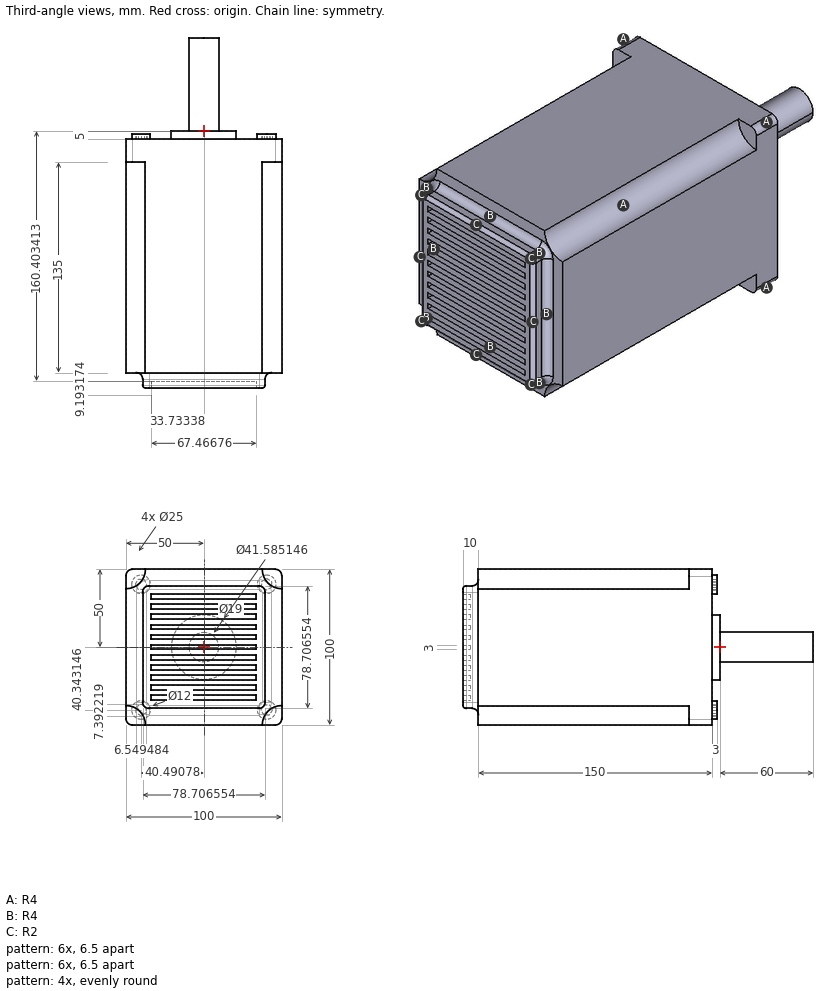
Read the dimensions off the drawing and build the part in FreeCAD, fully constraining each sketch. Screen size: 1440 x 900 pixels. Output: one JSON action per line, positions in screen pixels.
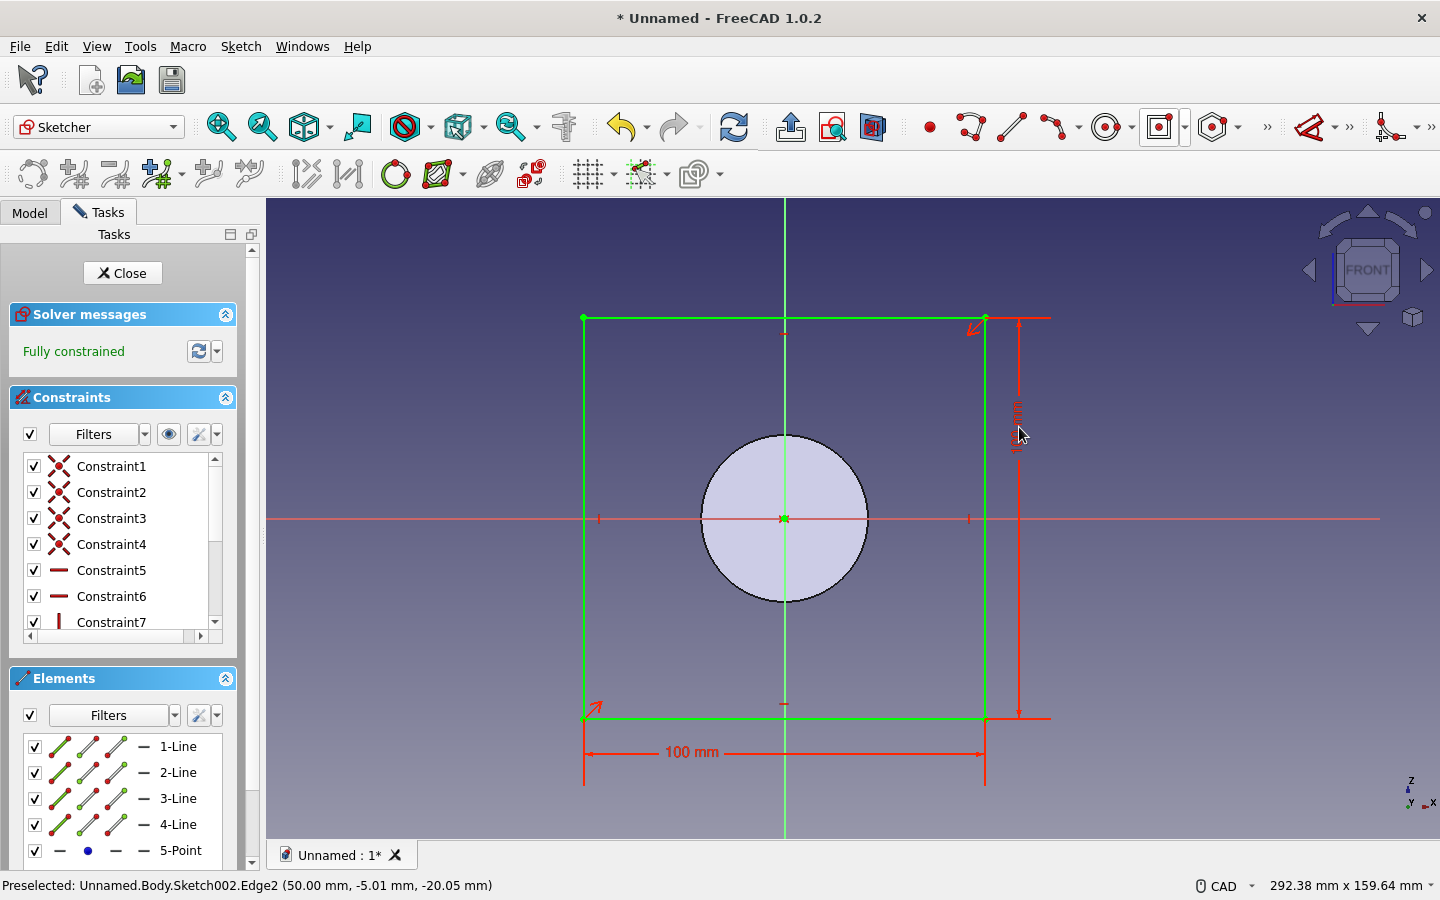
{"action": "left_click", "coordinate": [123, 273]}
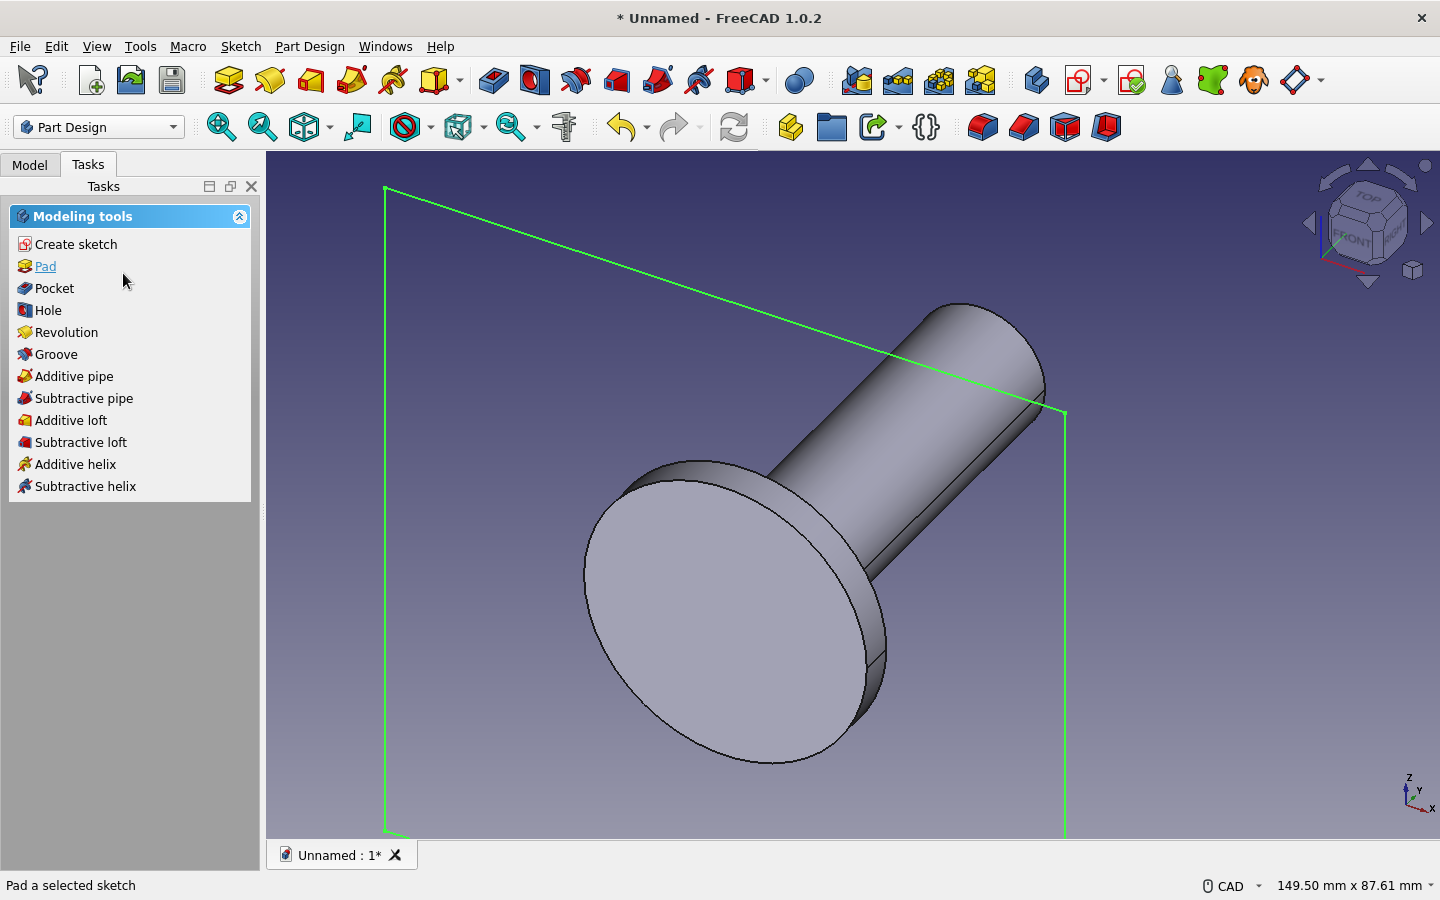
{"action": "left_click", "coordinate": [229, 80]}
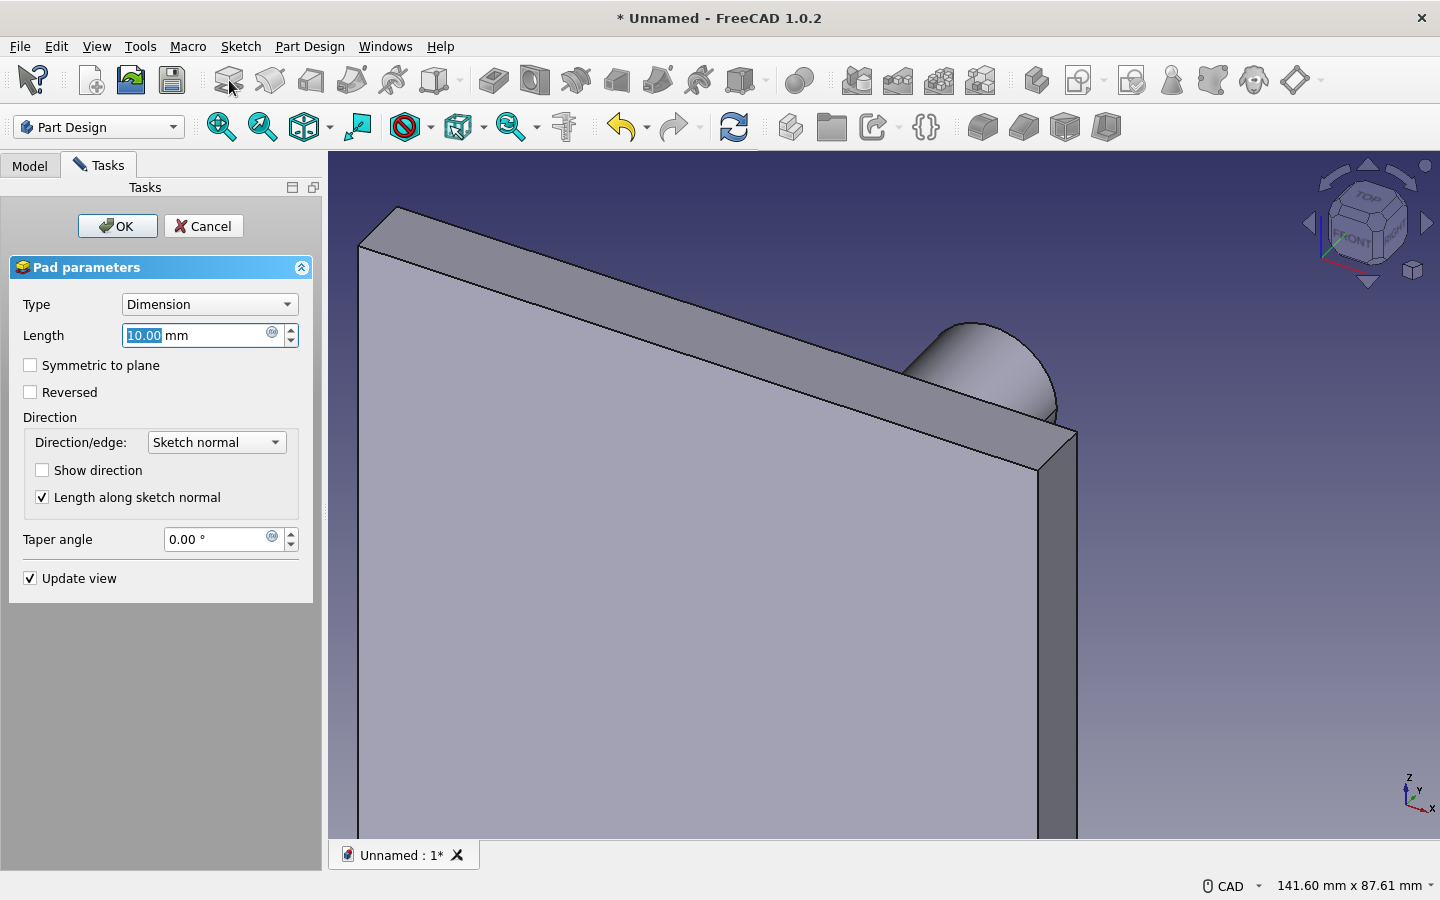
{"action": "type", "text": "150"}
{"action": "key", "text": "Tab"}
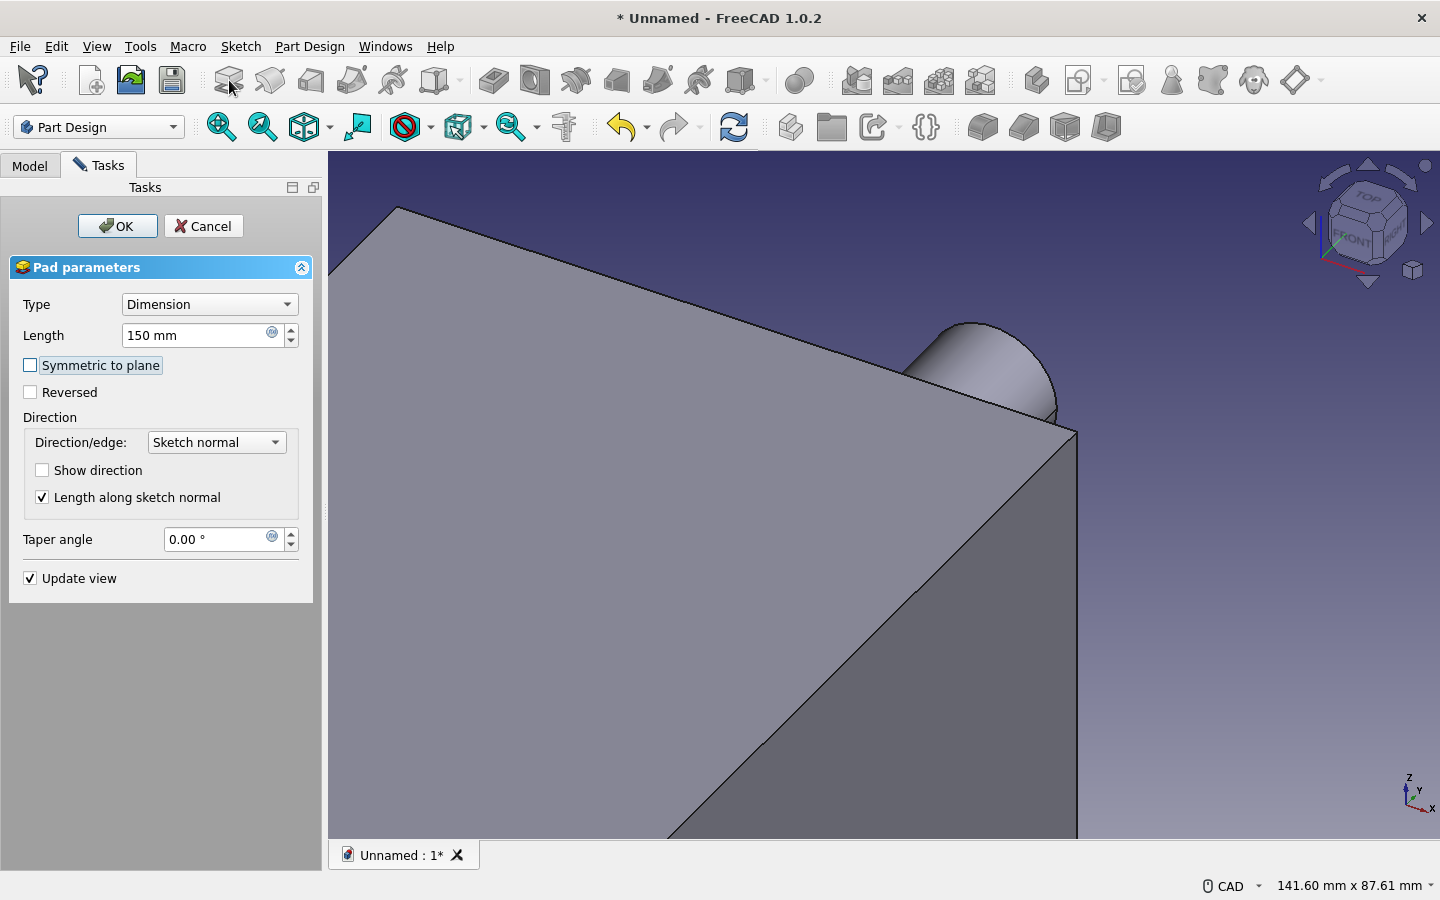
{"action": "left_click", "coordinate": [118, 226]}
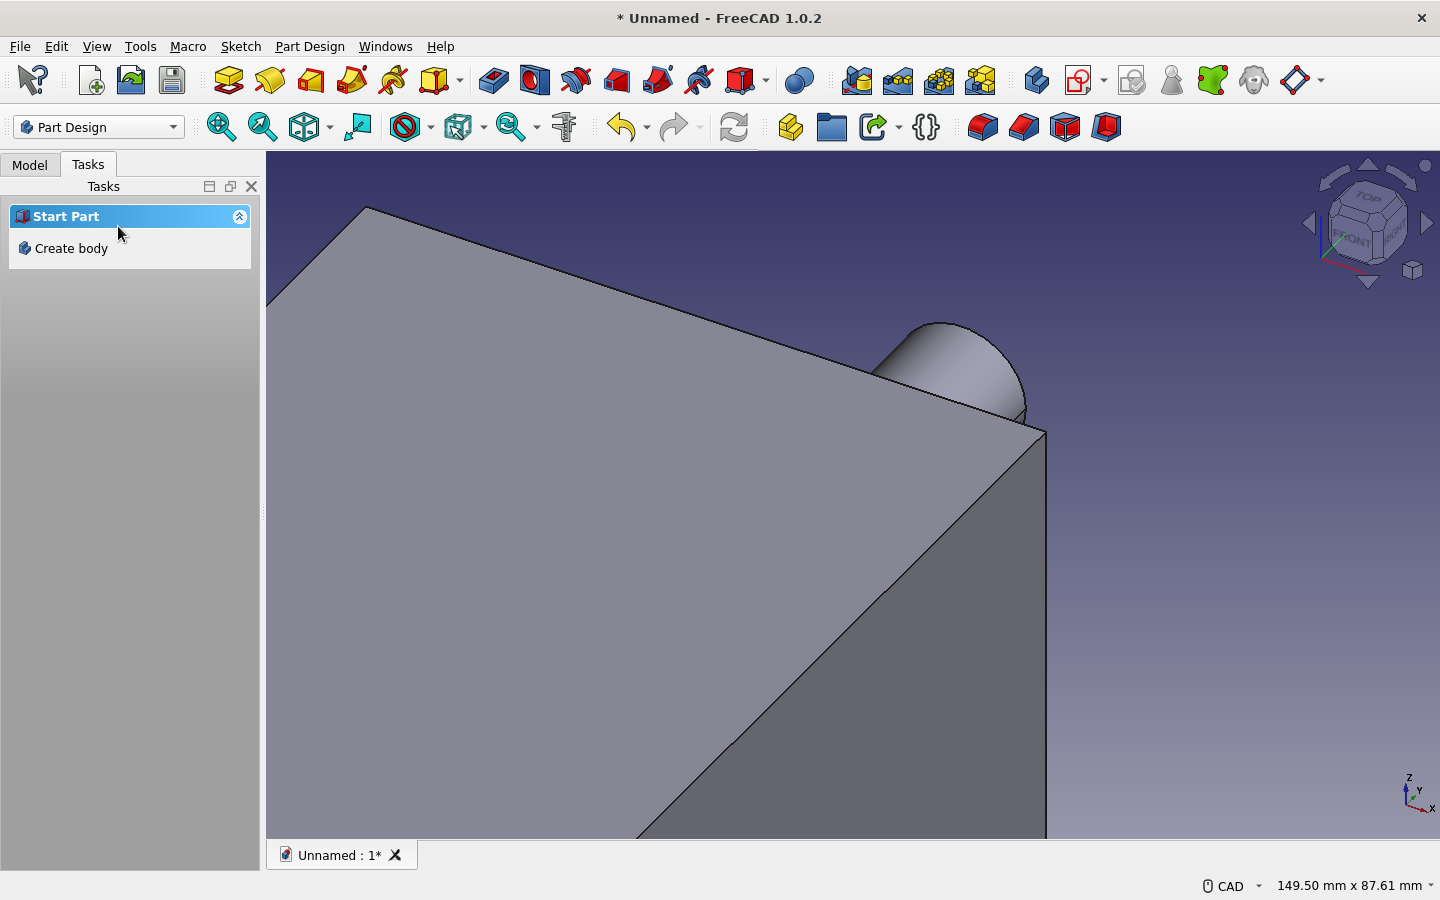
{"action": "left_click", "coordinate": [222, 128]}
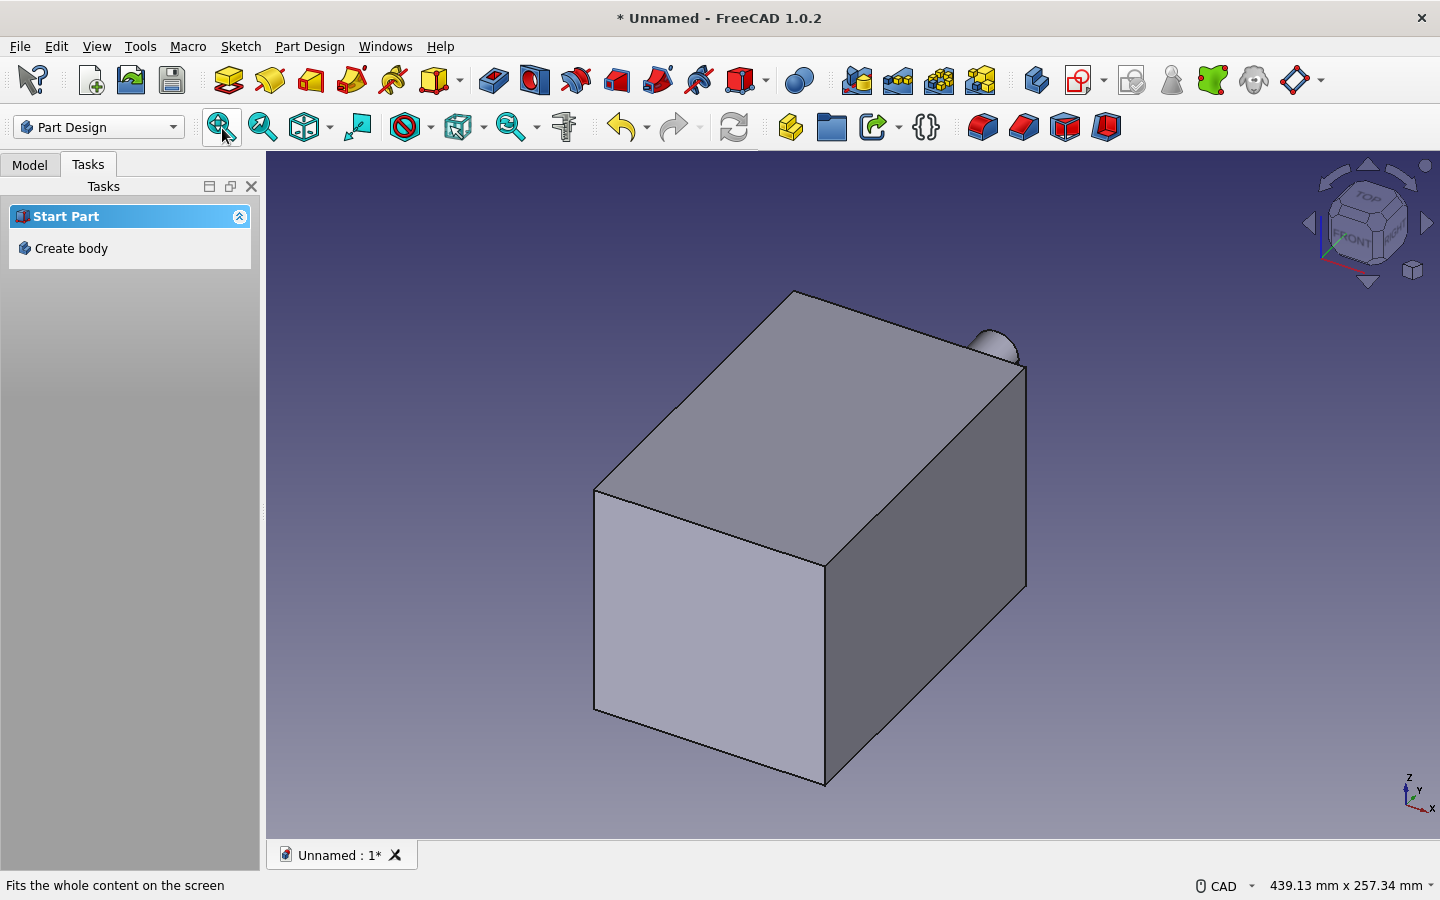
{"action": "left_click", "coordinate": [709, 637]}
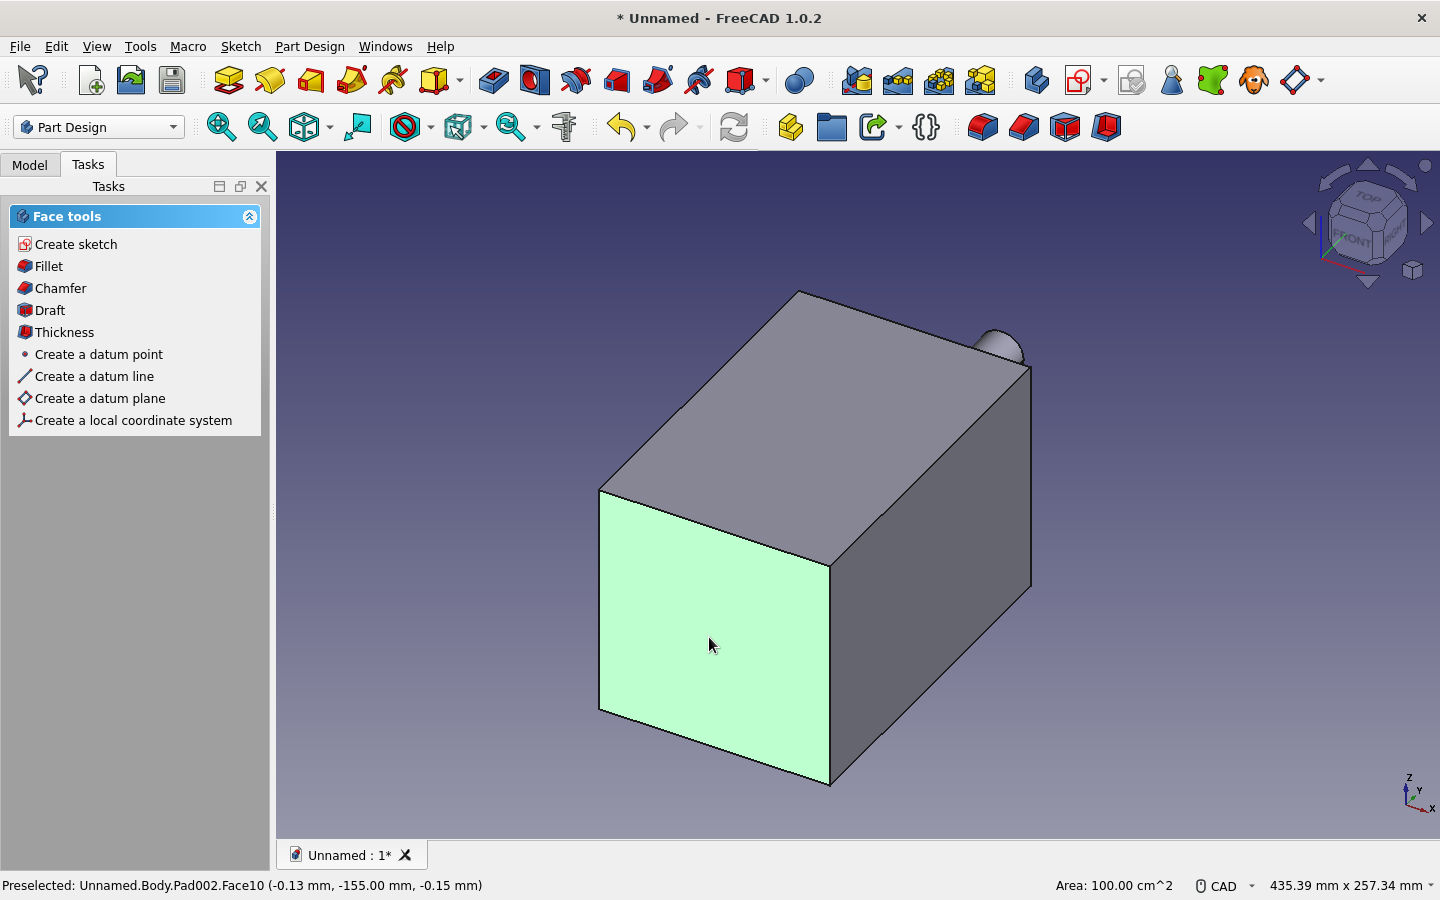
{"action": "left_click", "coordinate": [1078, 80]}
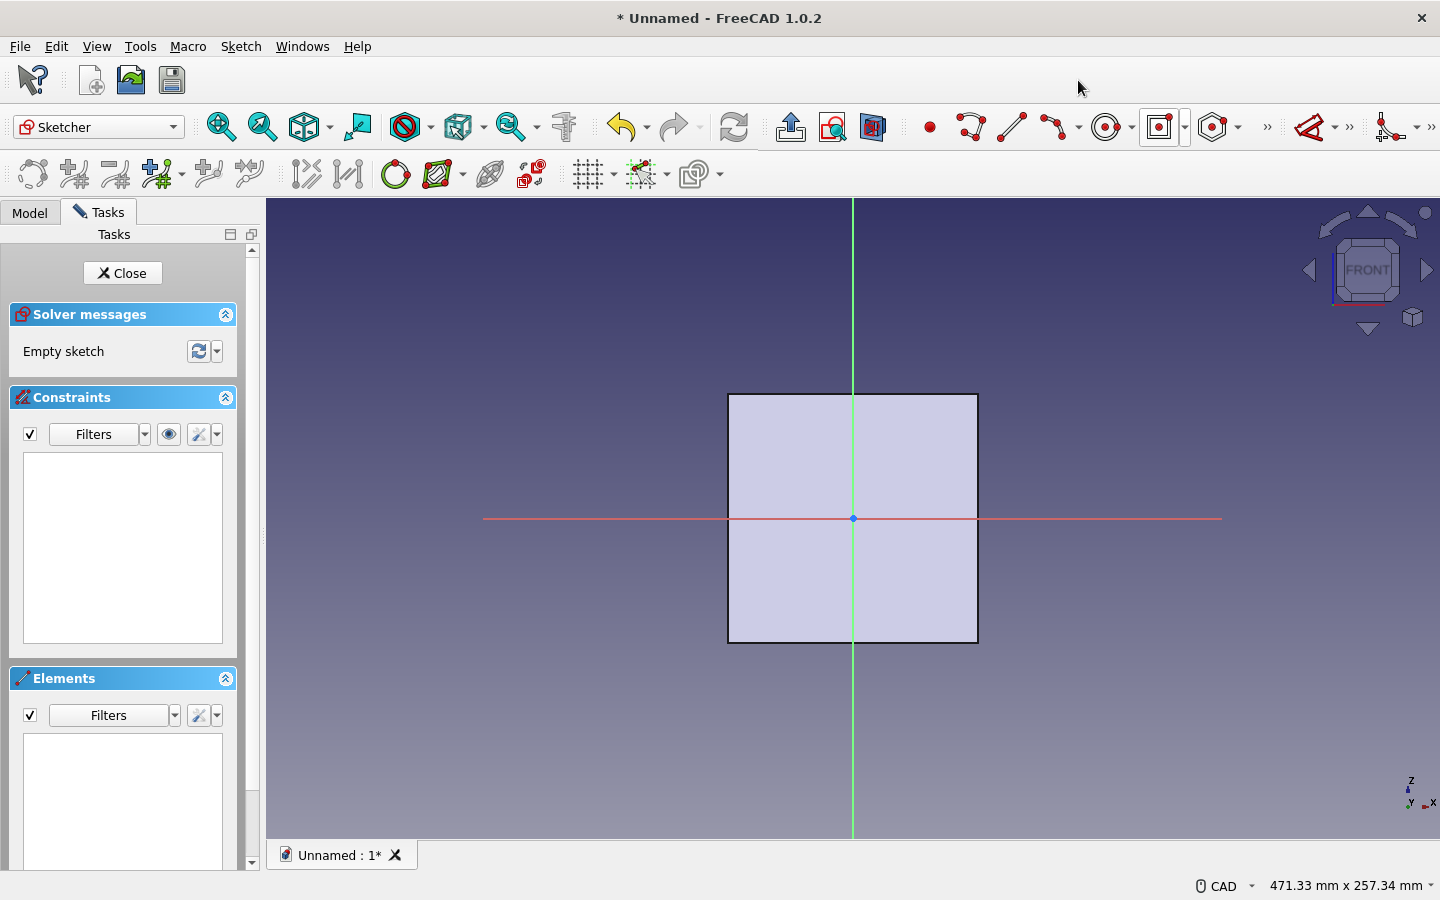
{"action": "left_click", "coordinate": [1106, 128]}